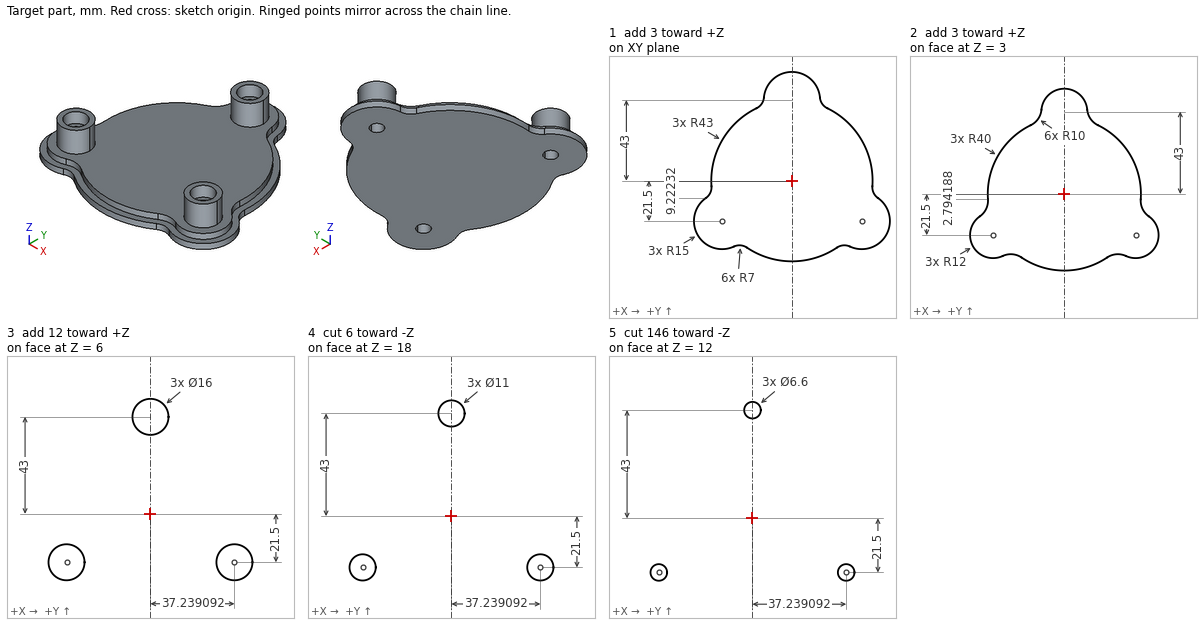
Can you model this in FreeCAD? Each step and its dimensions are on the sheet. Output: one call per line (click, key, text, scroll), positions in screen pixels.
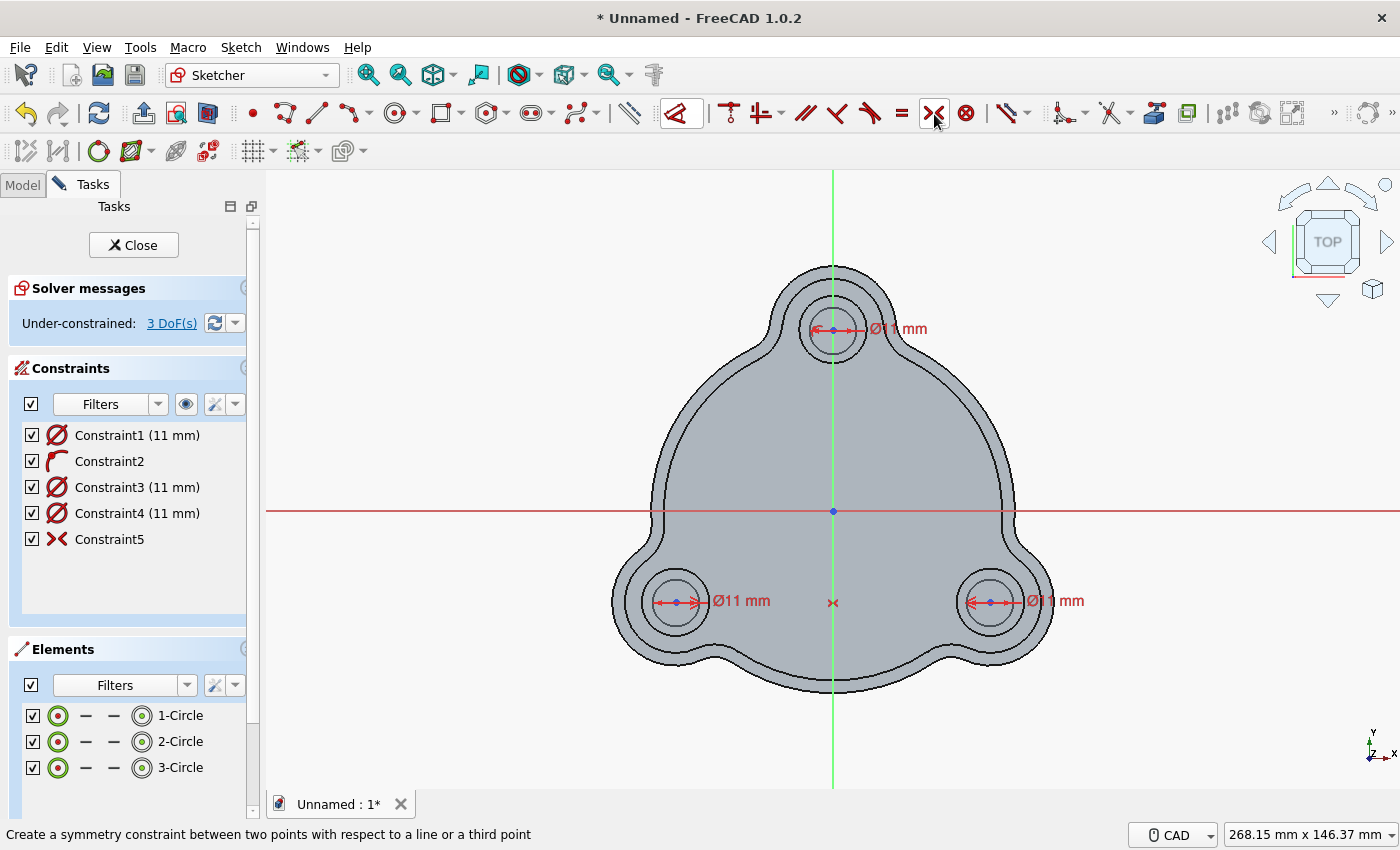
click(833, 331)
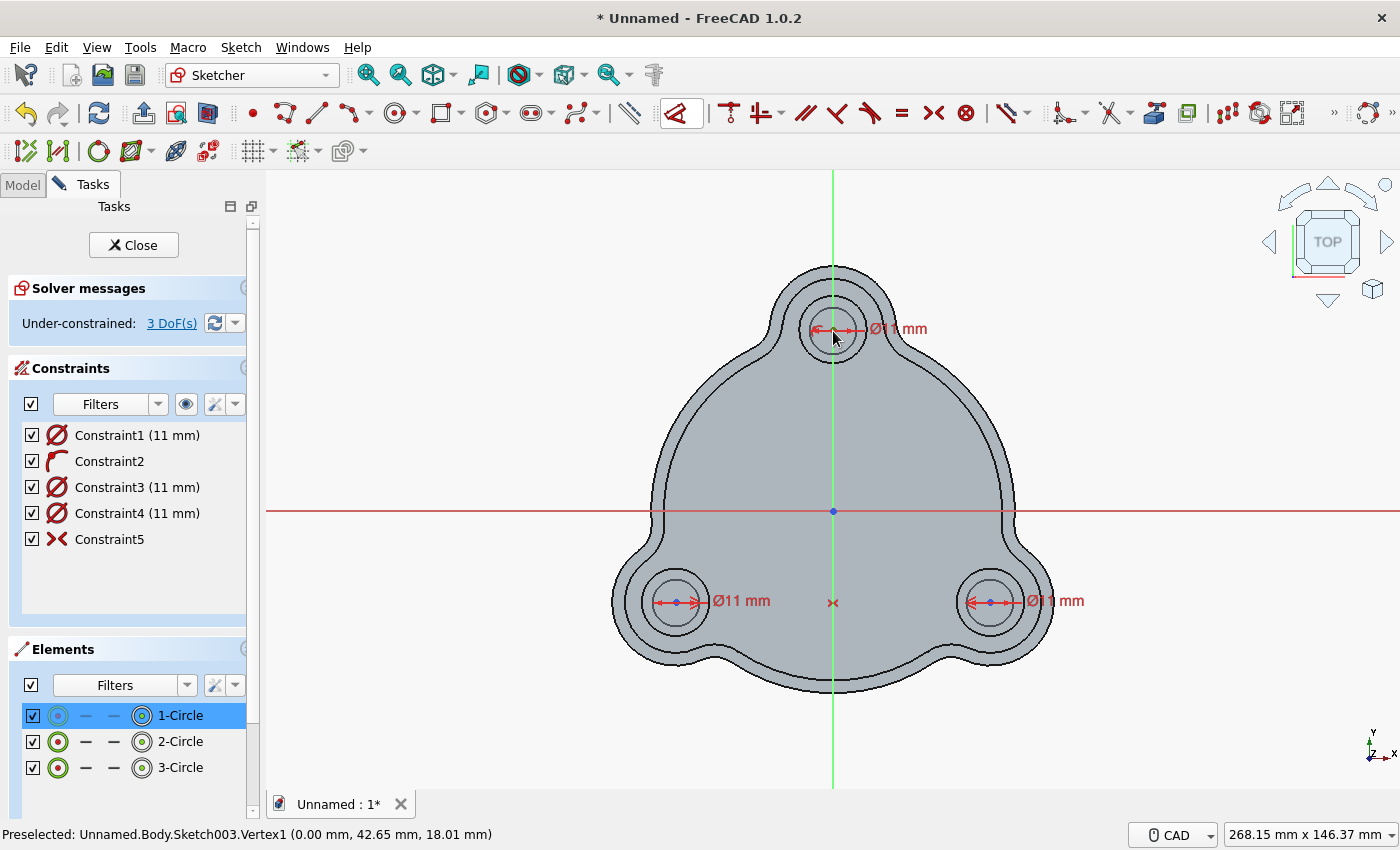
click(698, 114)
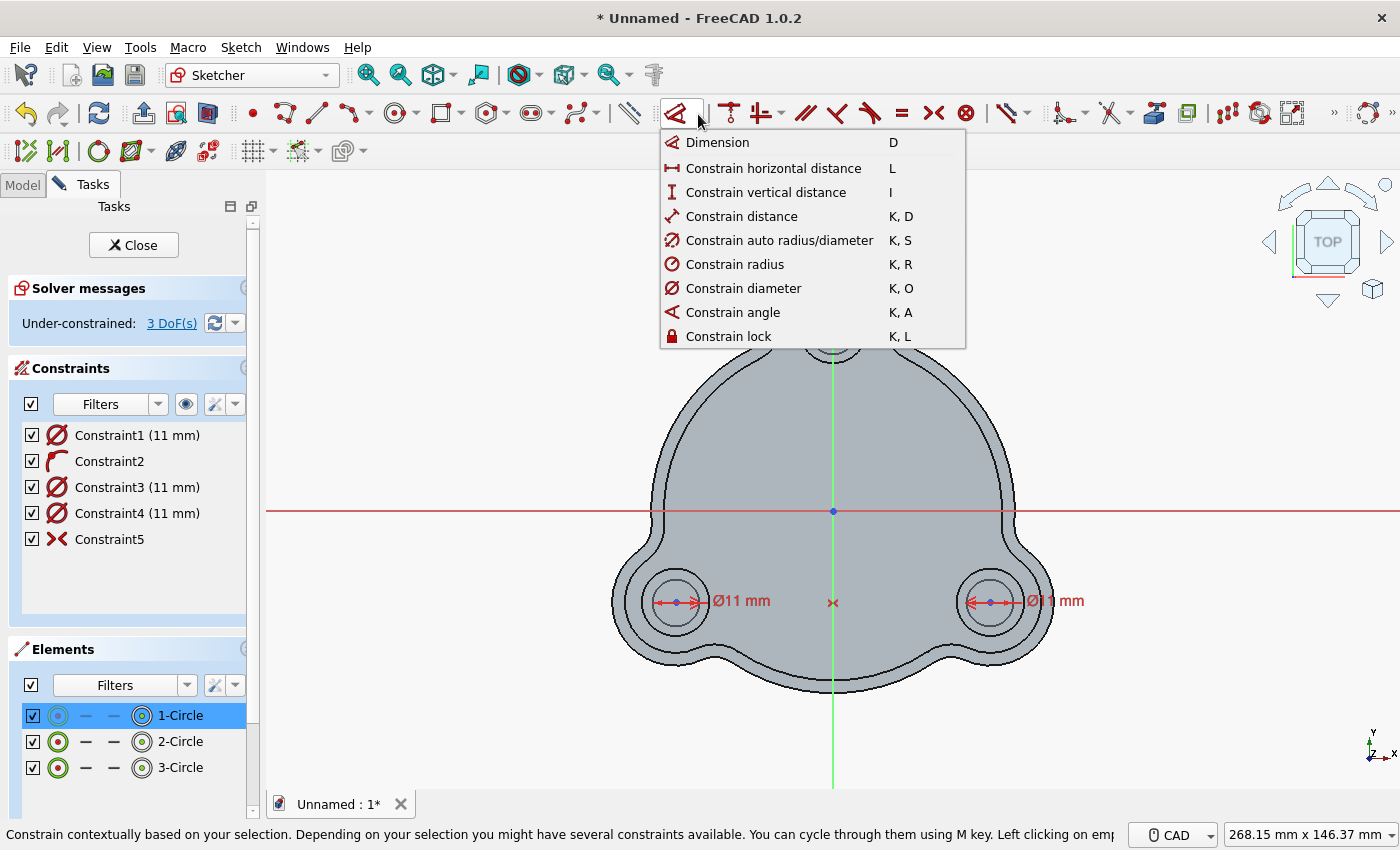
click(813, 192)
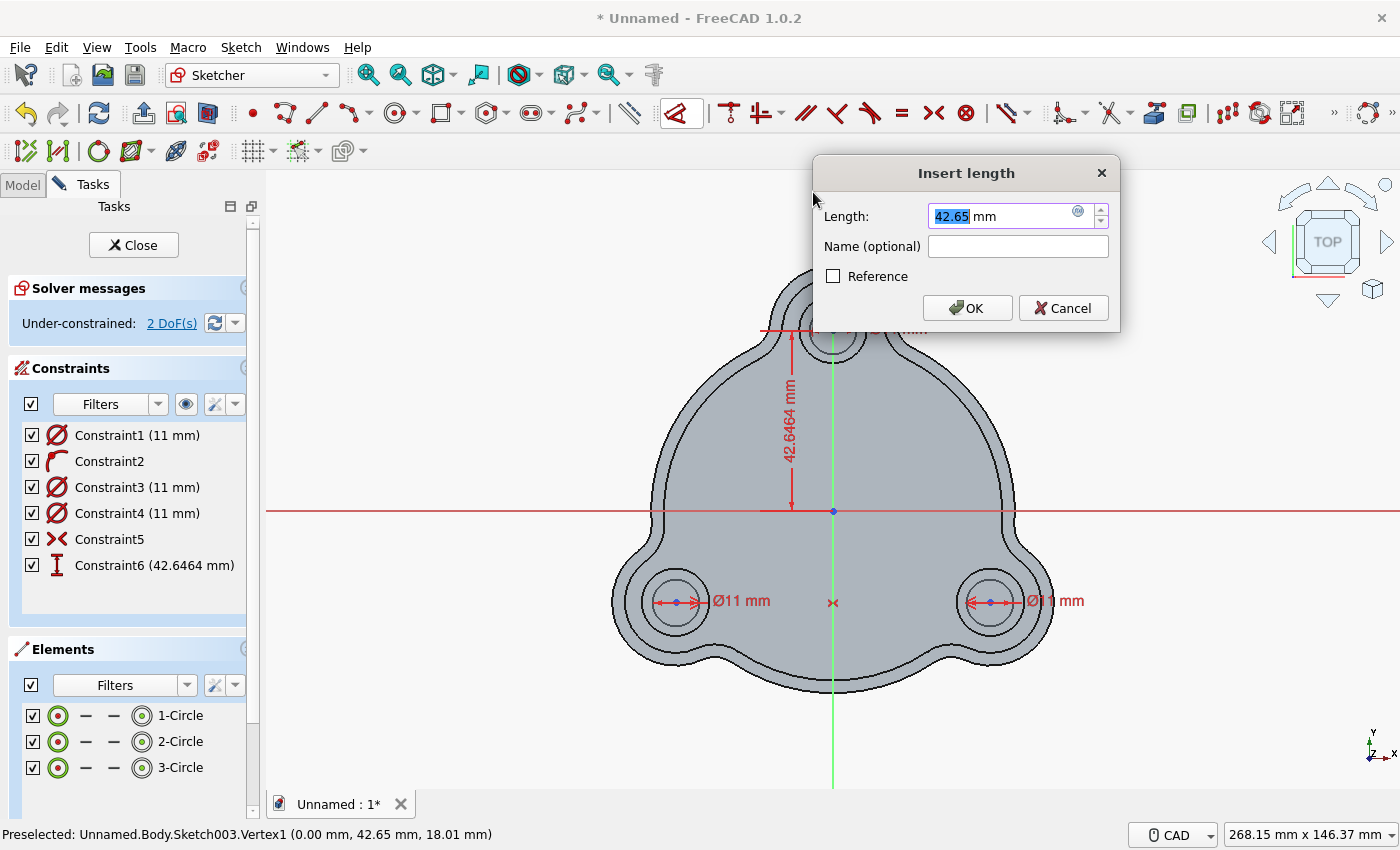
text(43)
key(Return)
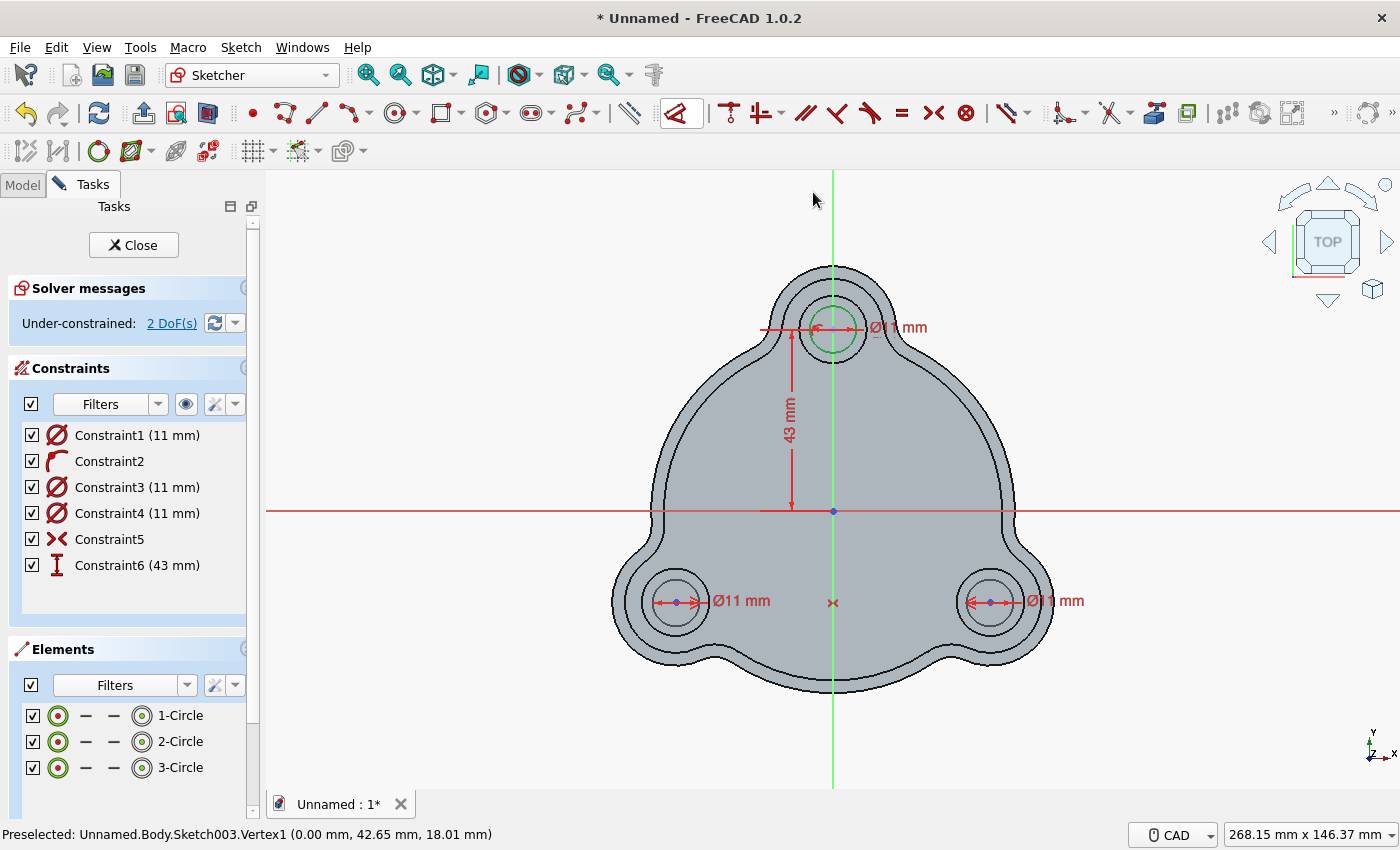
click(990, 603)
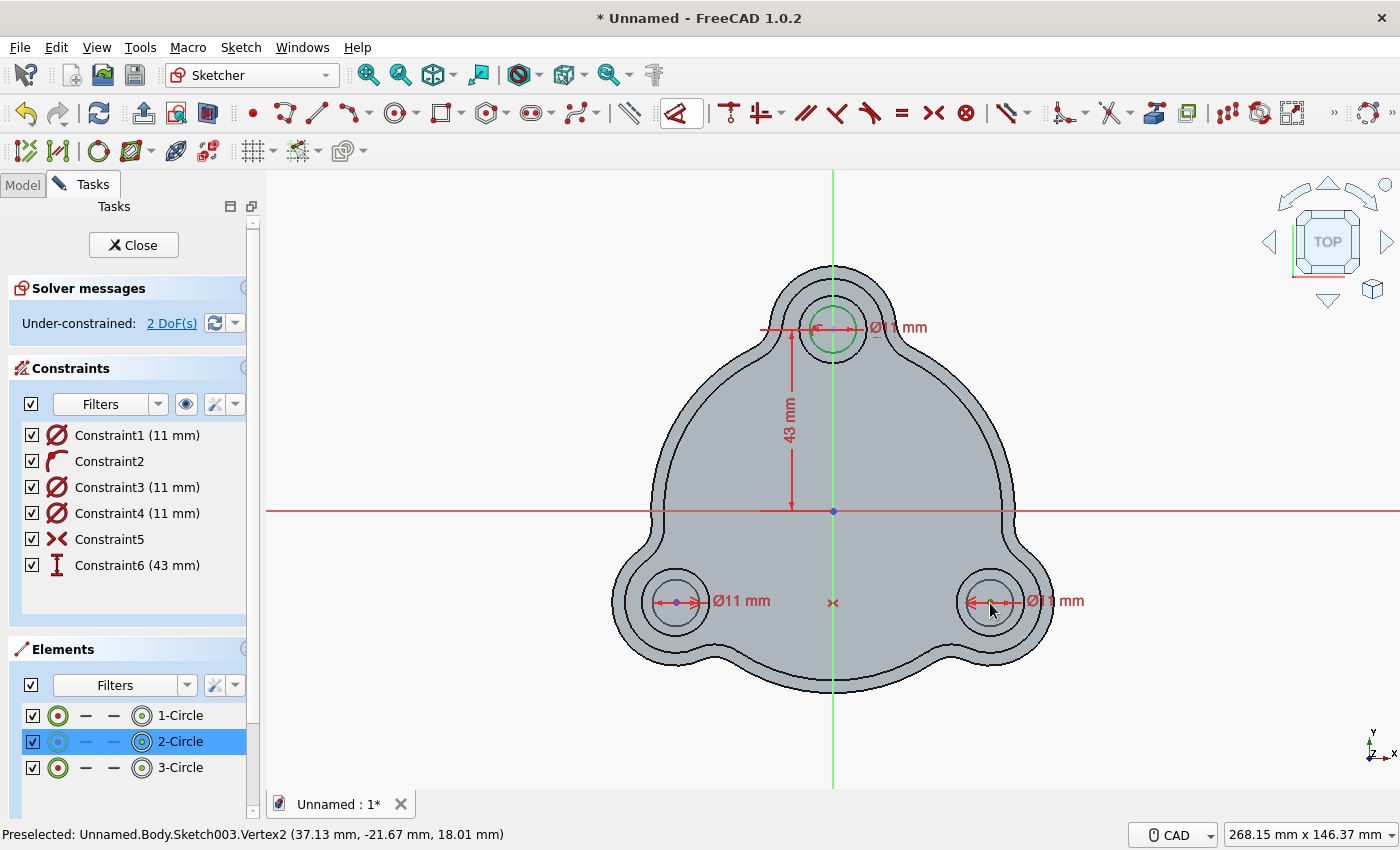
key(i)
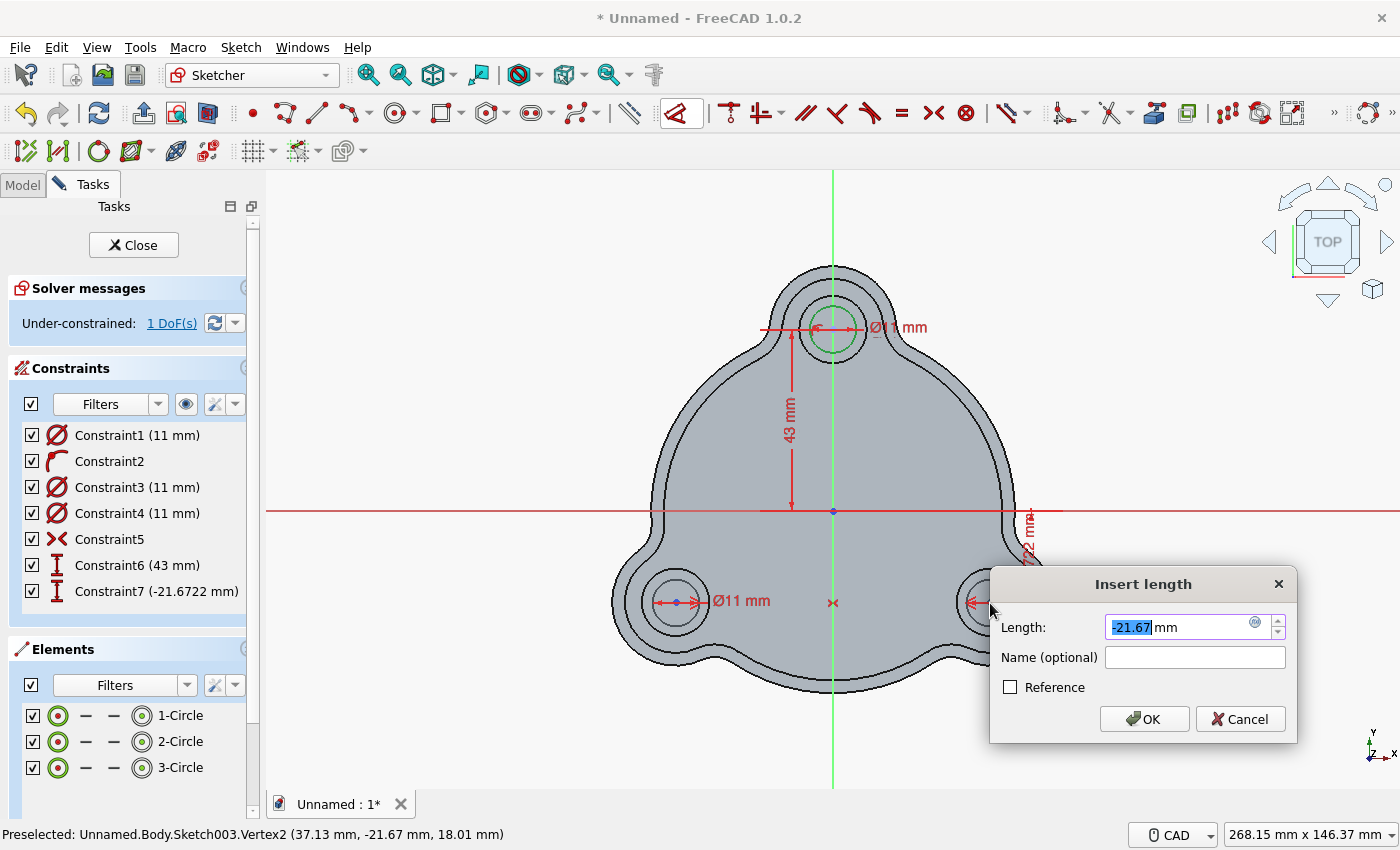
text(-21.5)
key(Return)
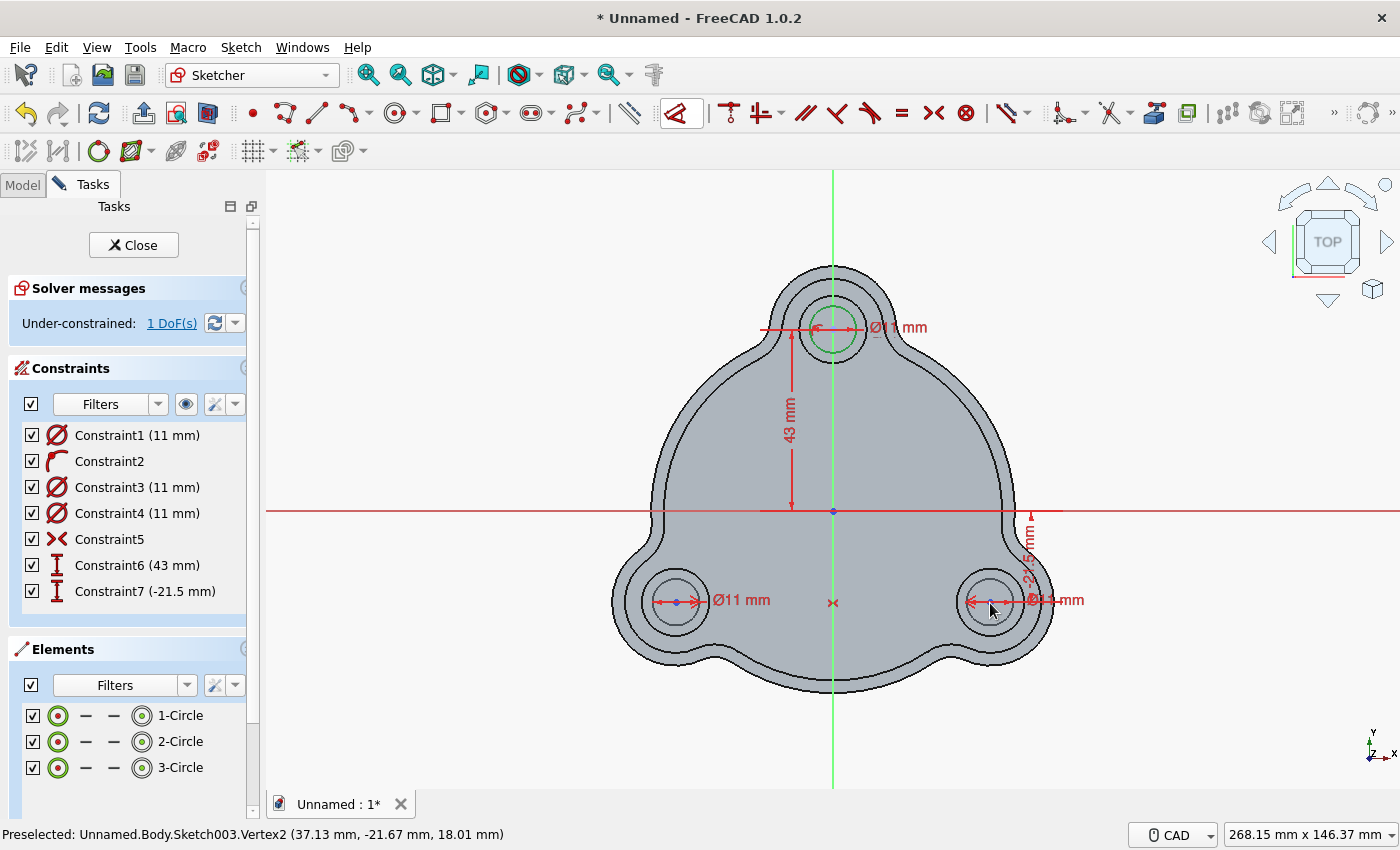
click(990, 602)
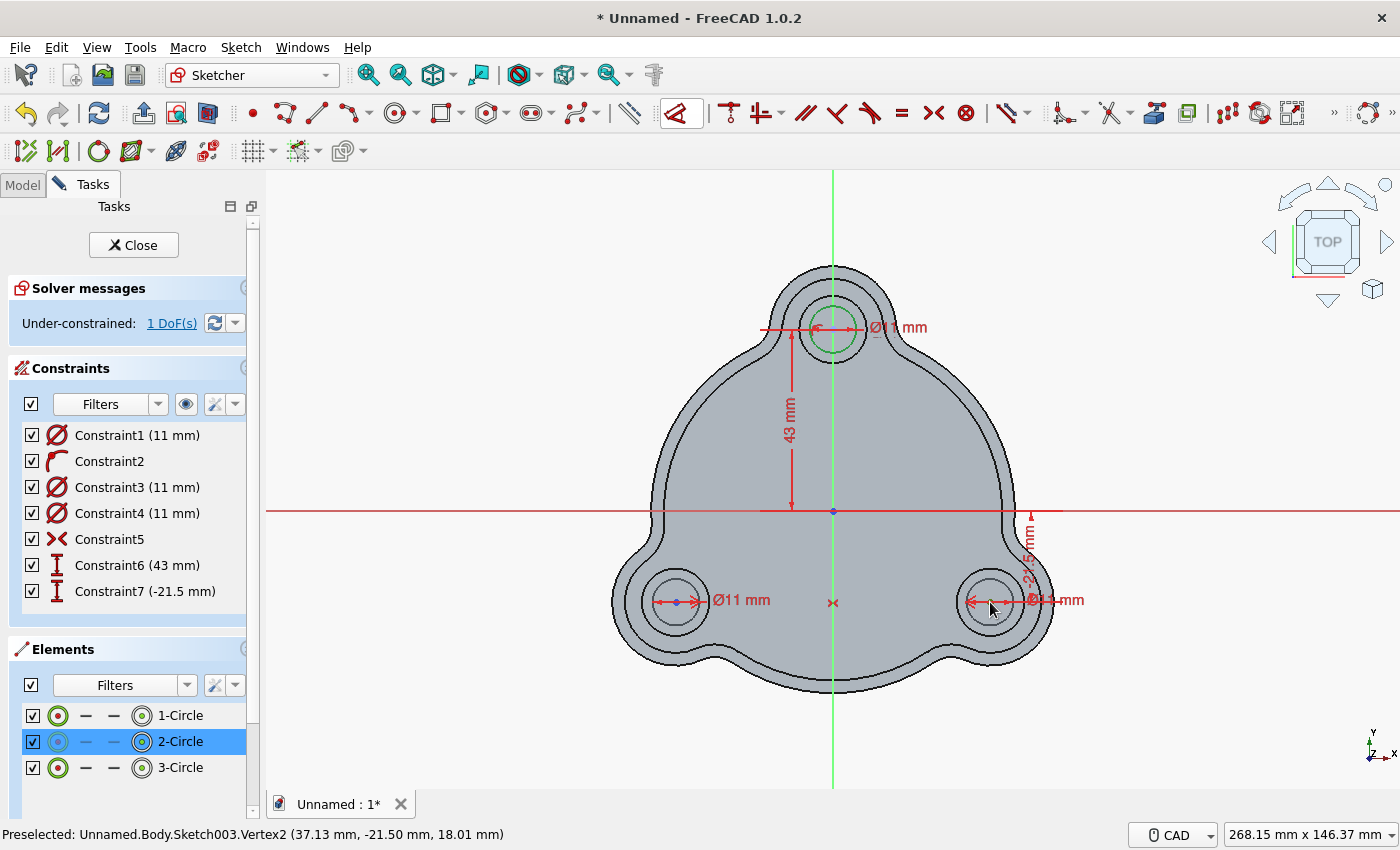
key(l)